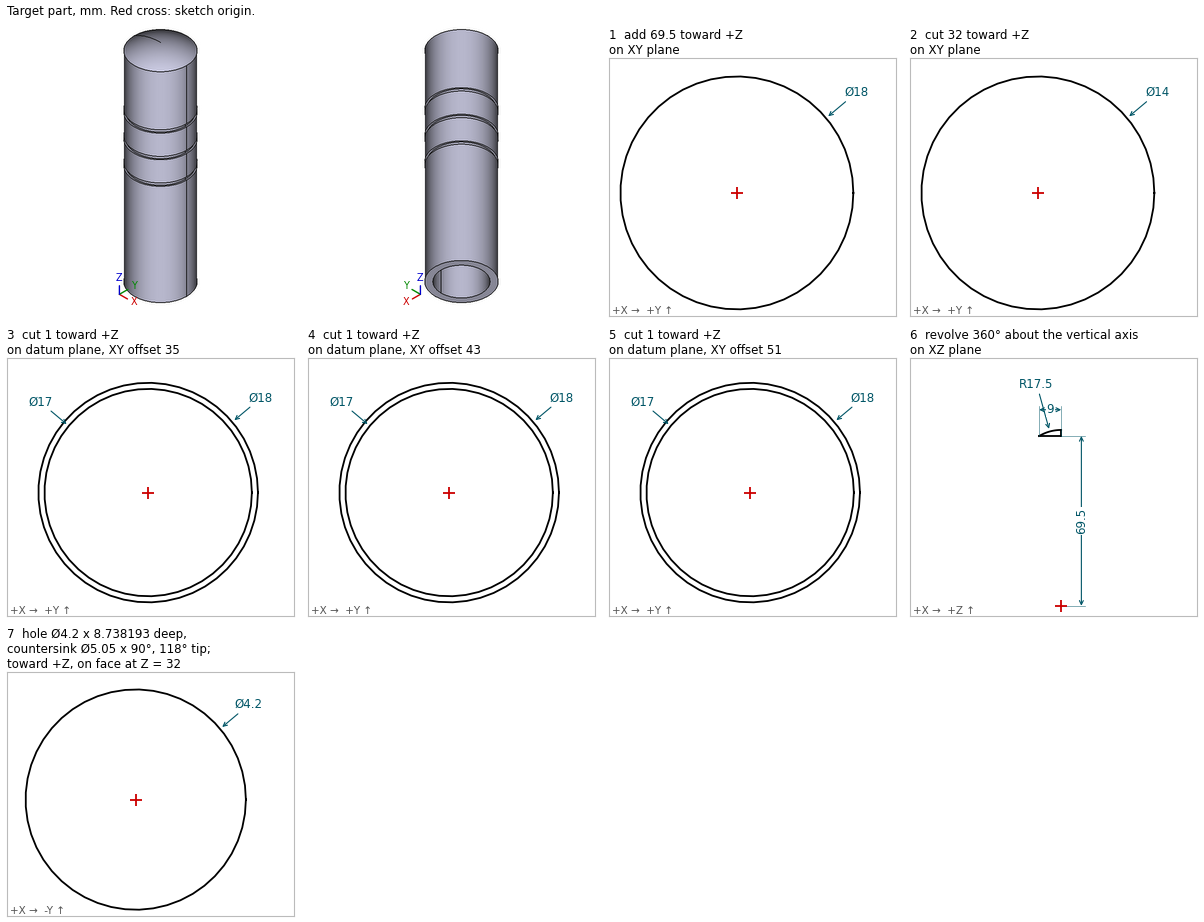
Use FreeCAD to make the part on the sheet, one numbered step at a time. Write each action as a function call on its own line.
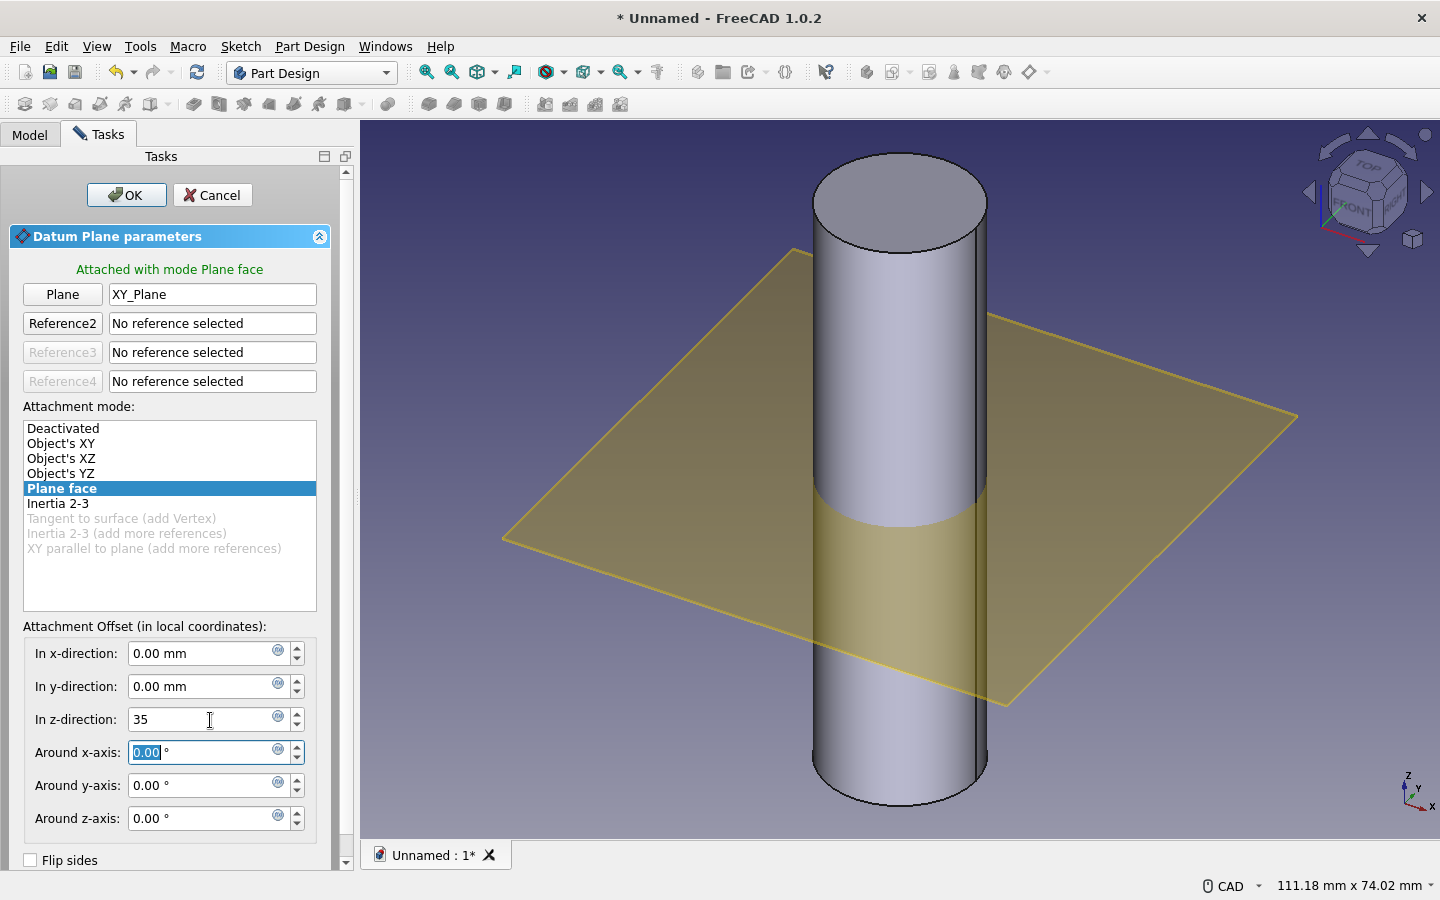
click(127, 195)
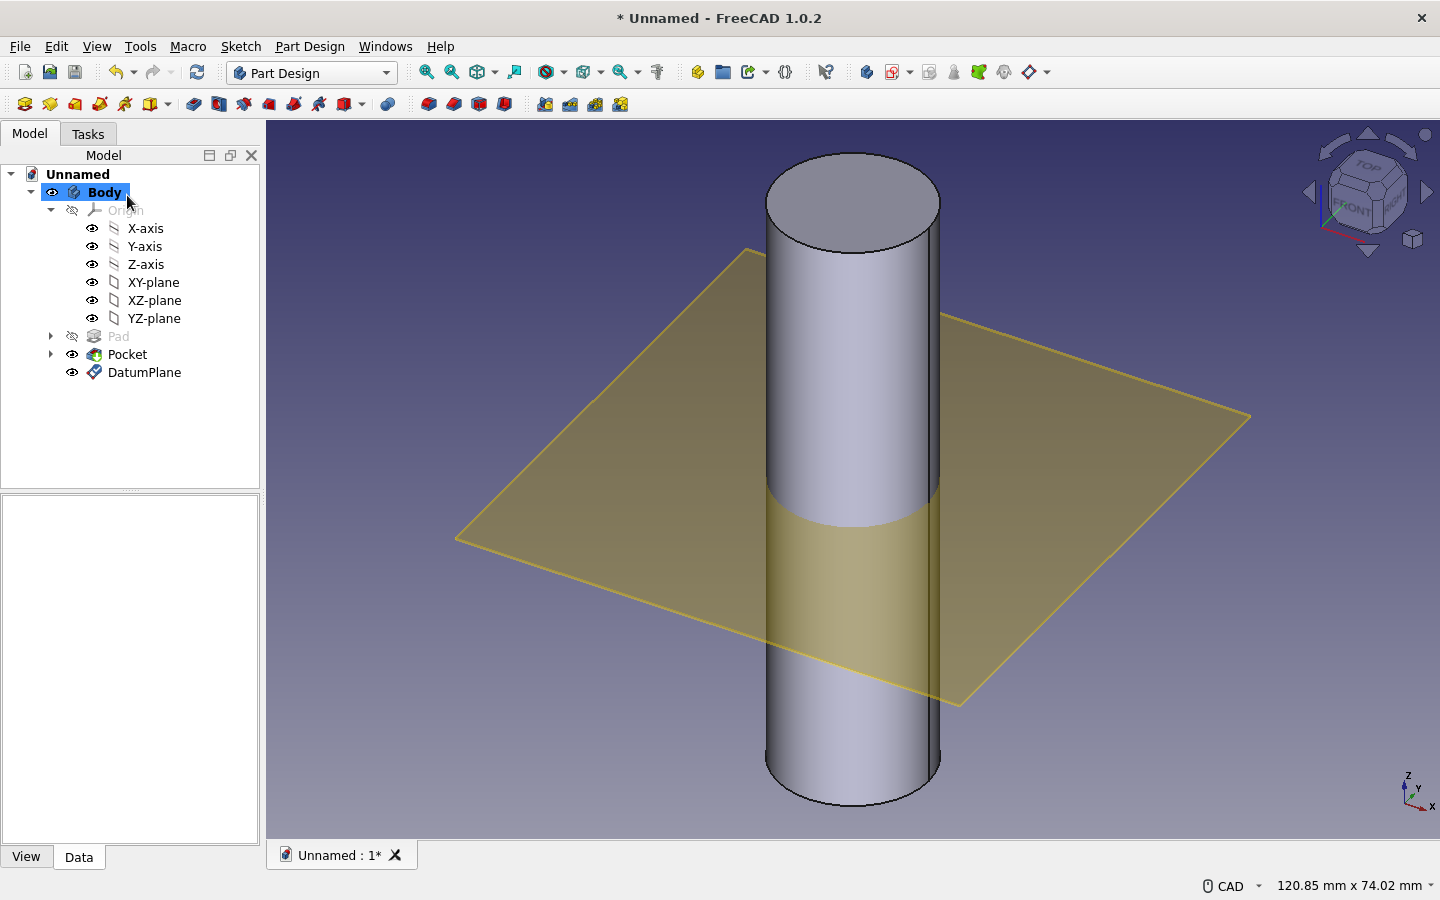
click(117, 372)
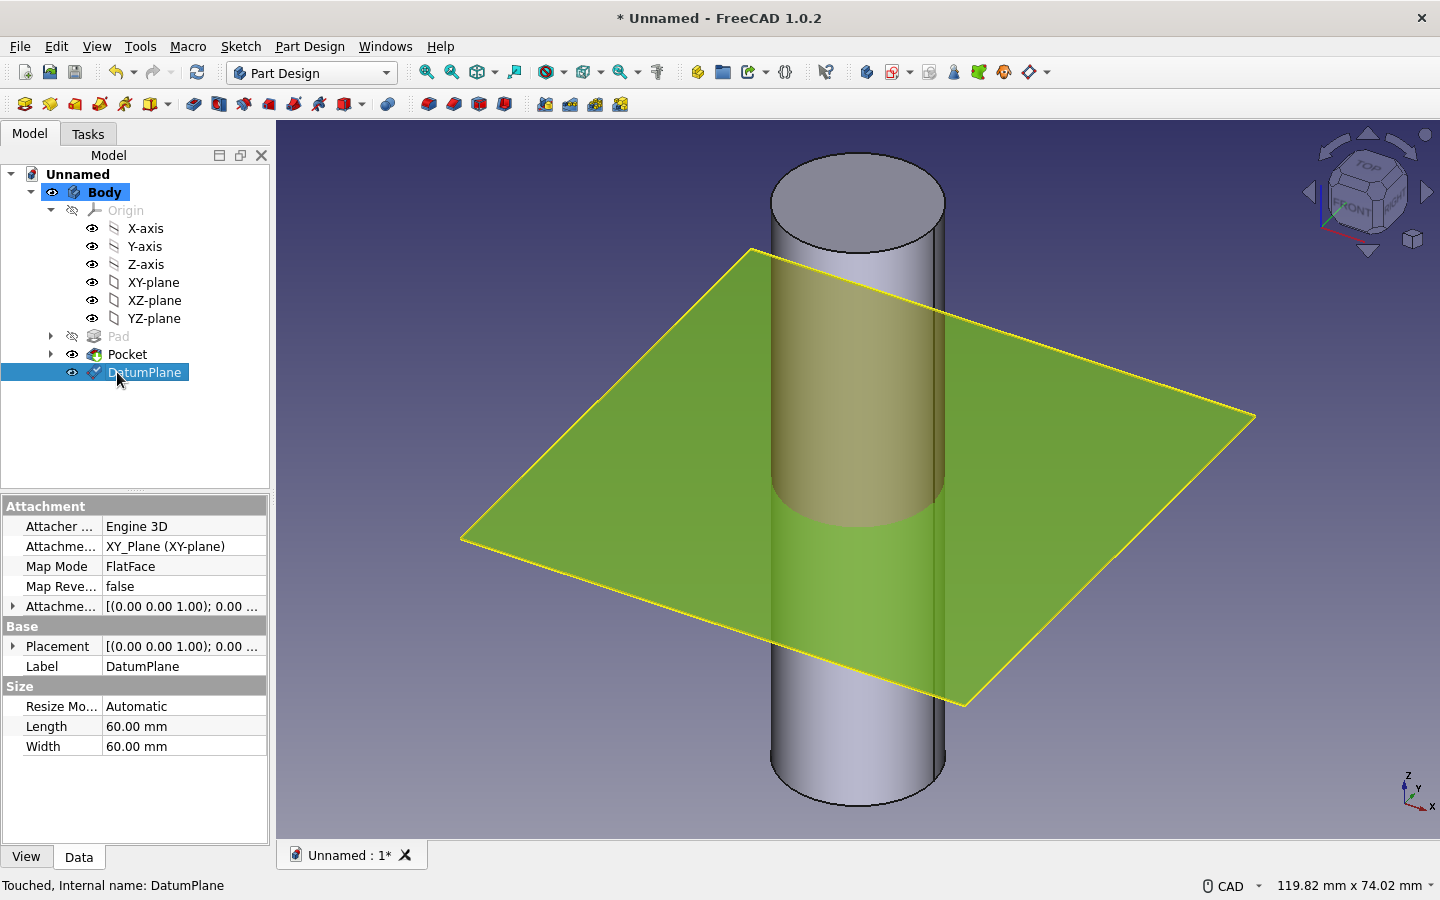
click(892, 72)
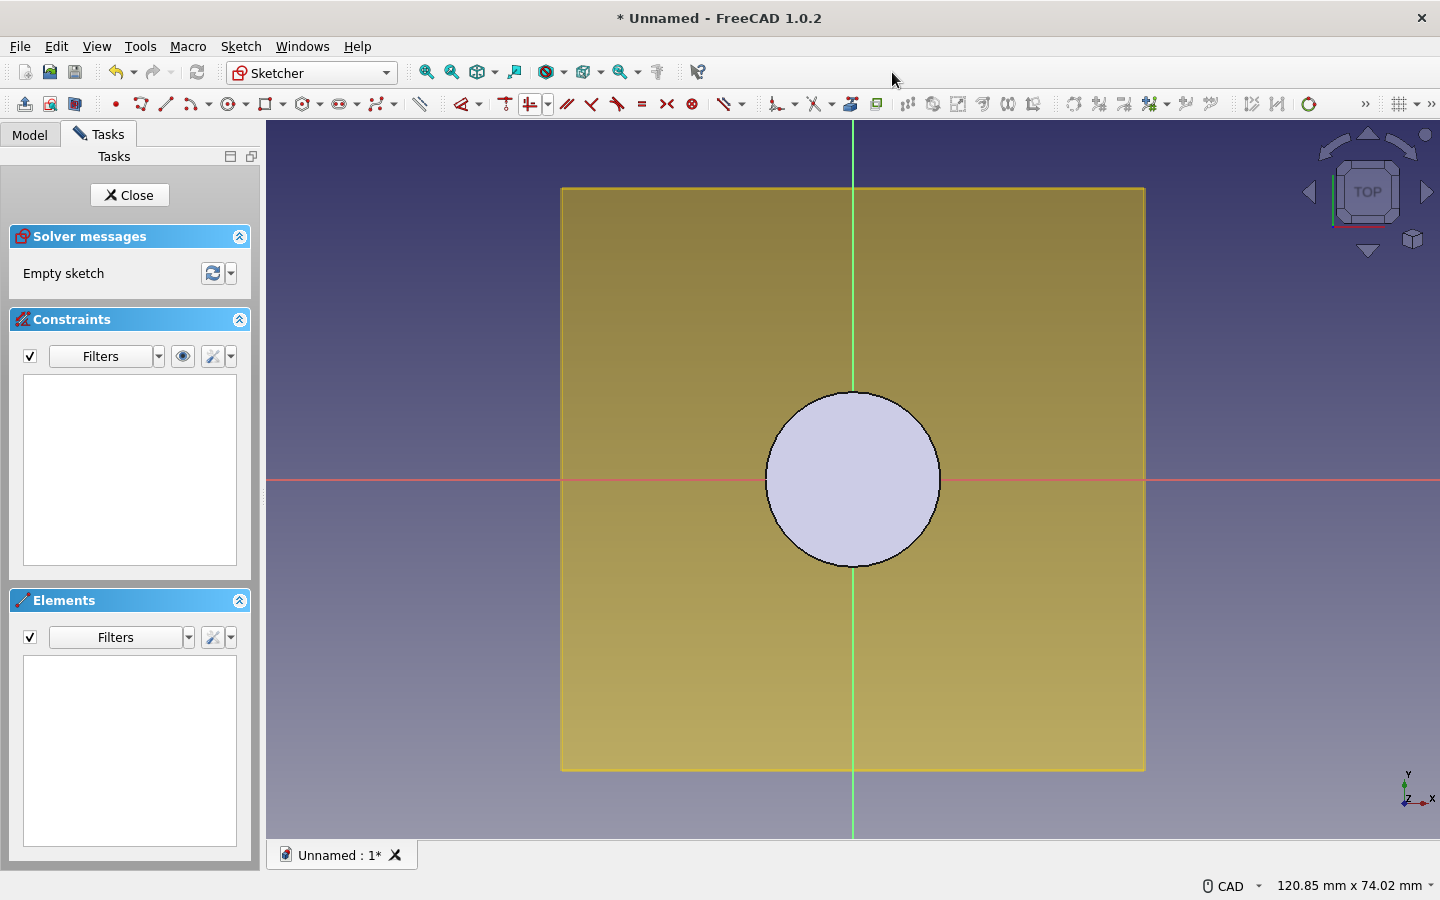
key(q)
key(s)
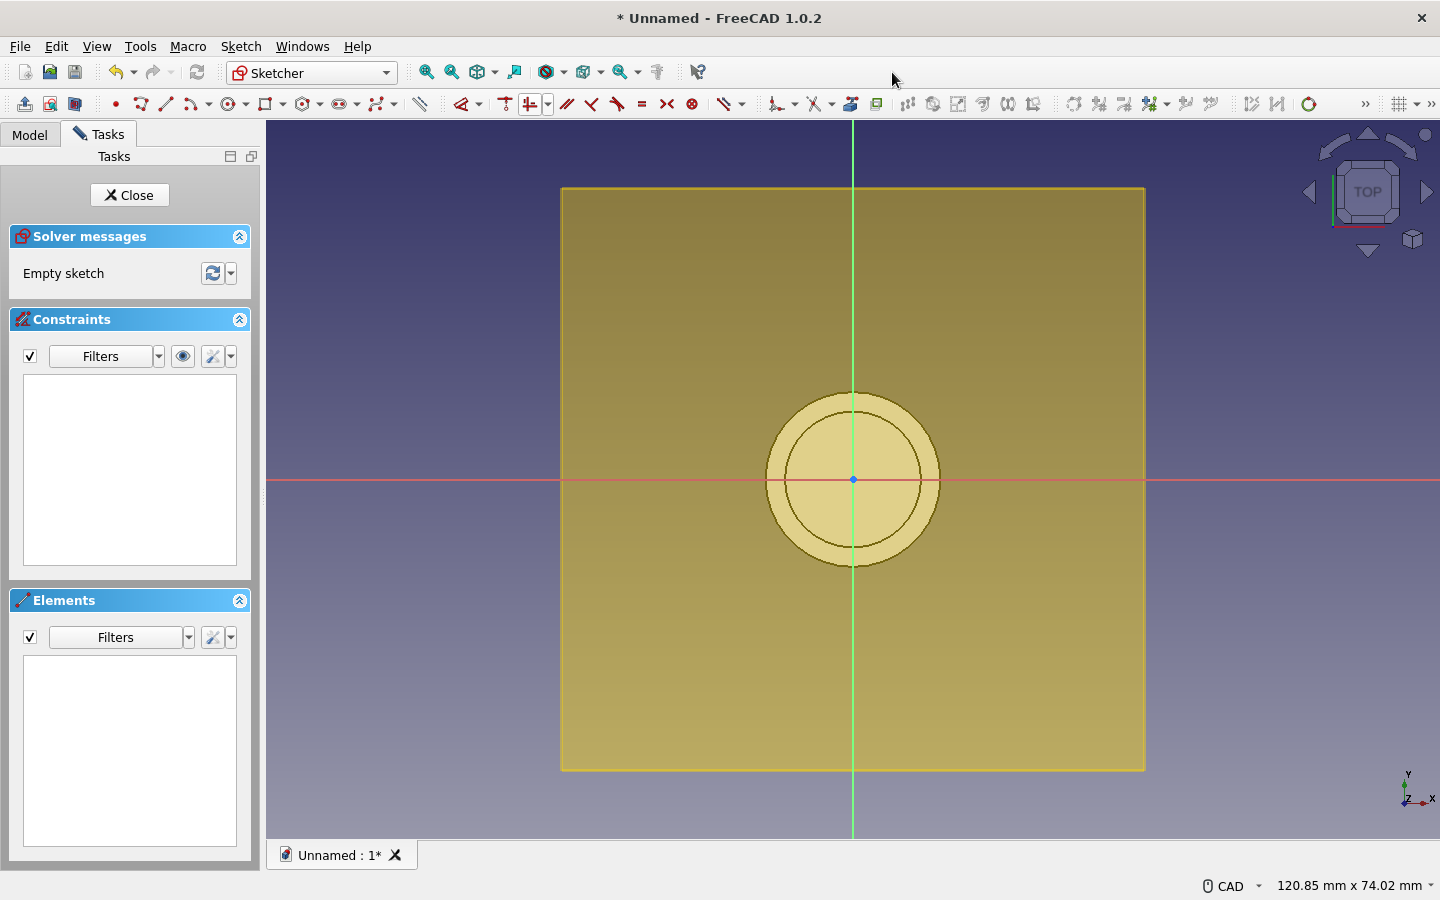
scroll(893, 480, up, 5)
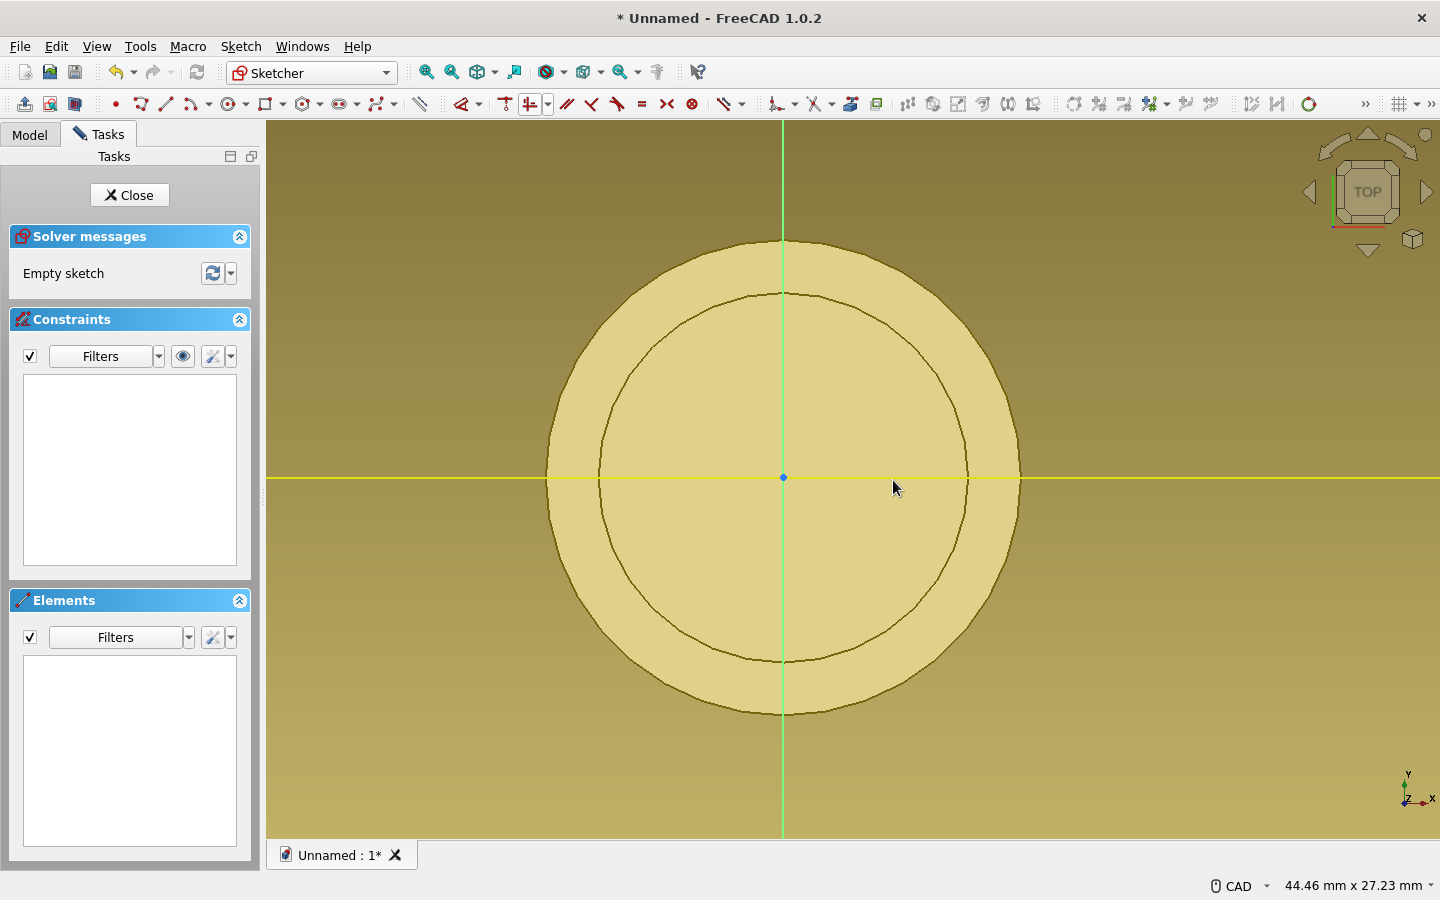
click(228, 104)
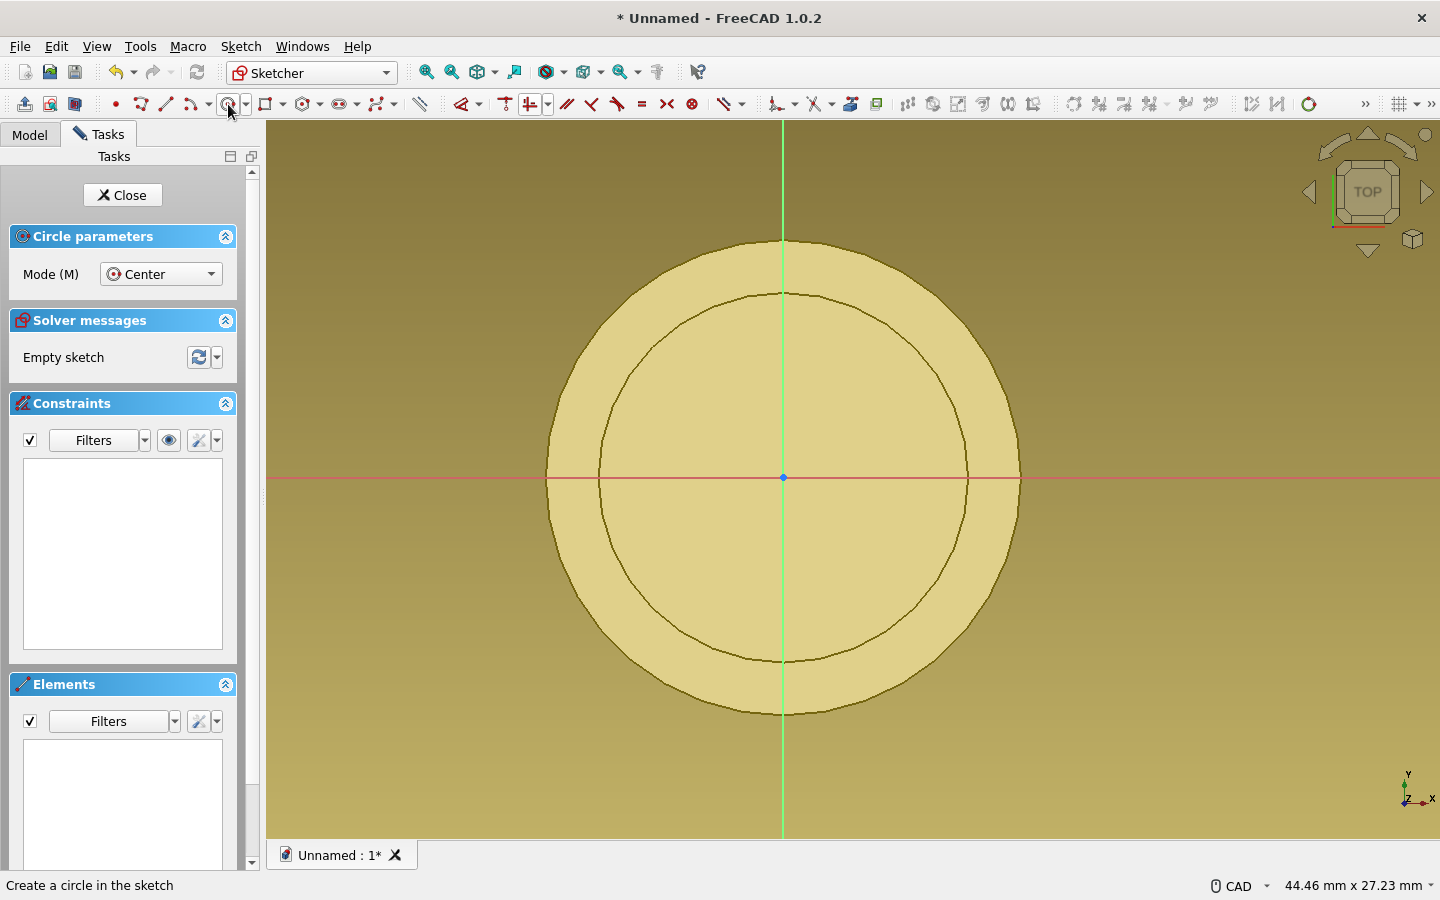
click(783, 478)
click(951, 310)